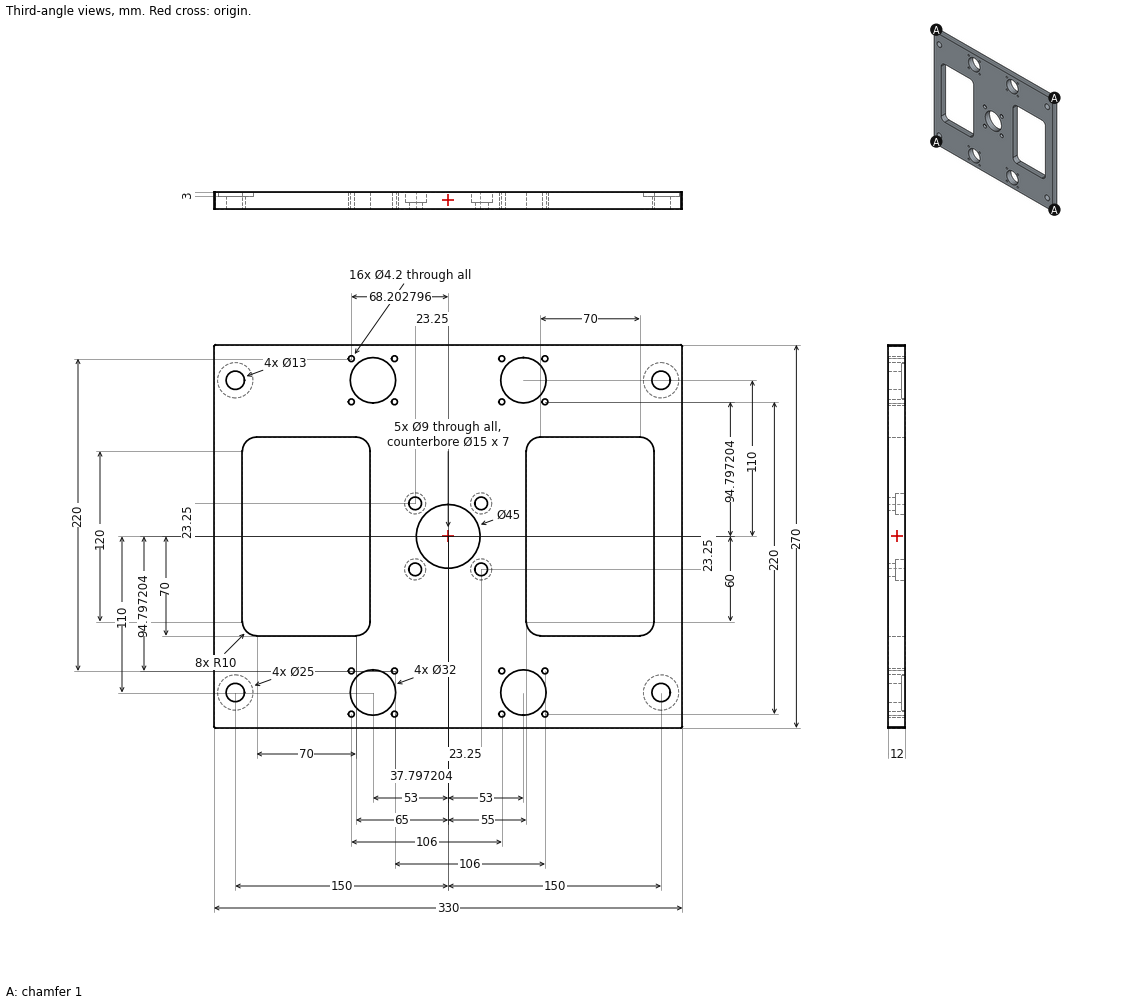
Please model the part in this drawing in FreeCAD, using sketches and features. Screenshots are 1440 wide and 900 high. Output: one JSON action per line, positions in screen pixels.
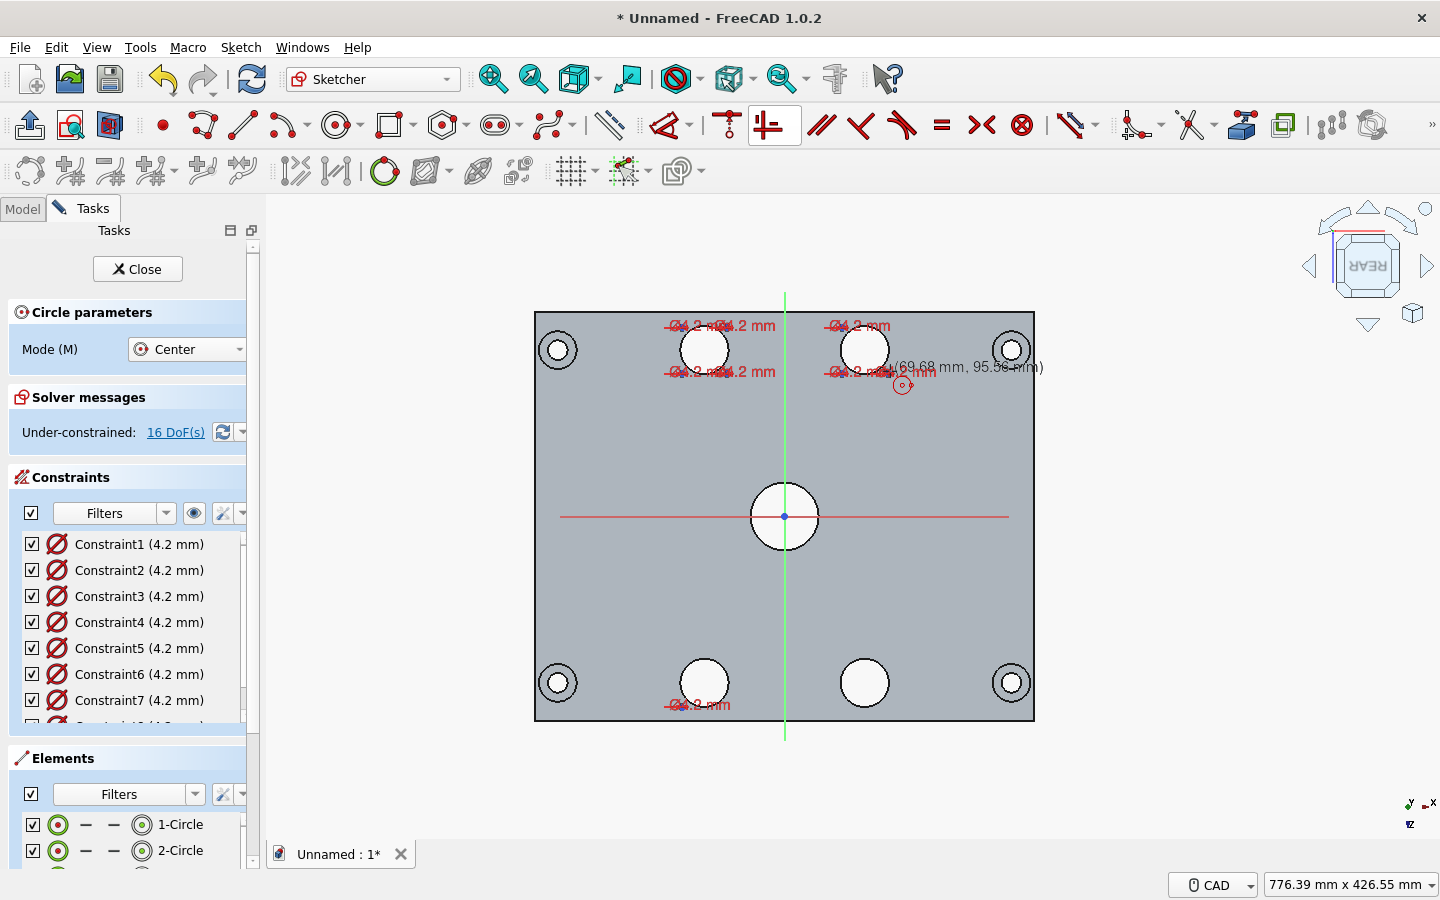
{"action": "scroll", "coordinate": [888, 327], "scroll_direction": "up", "scroll_amount": 10}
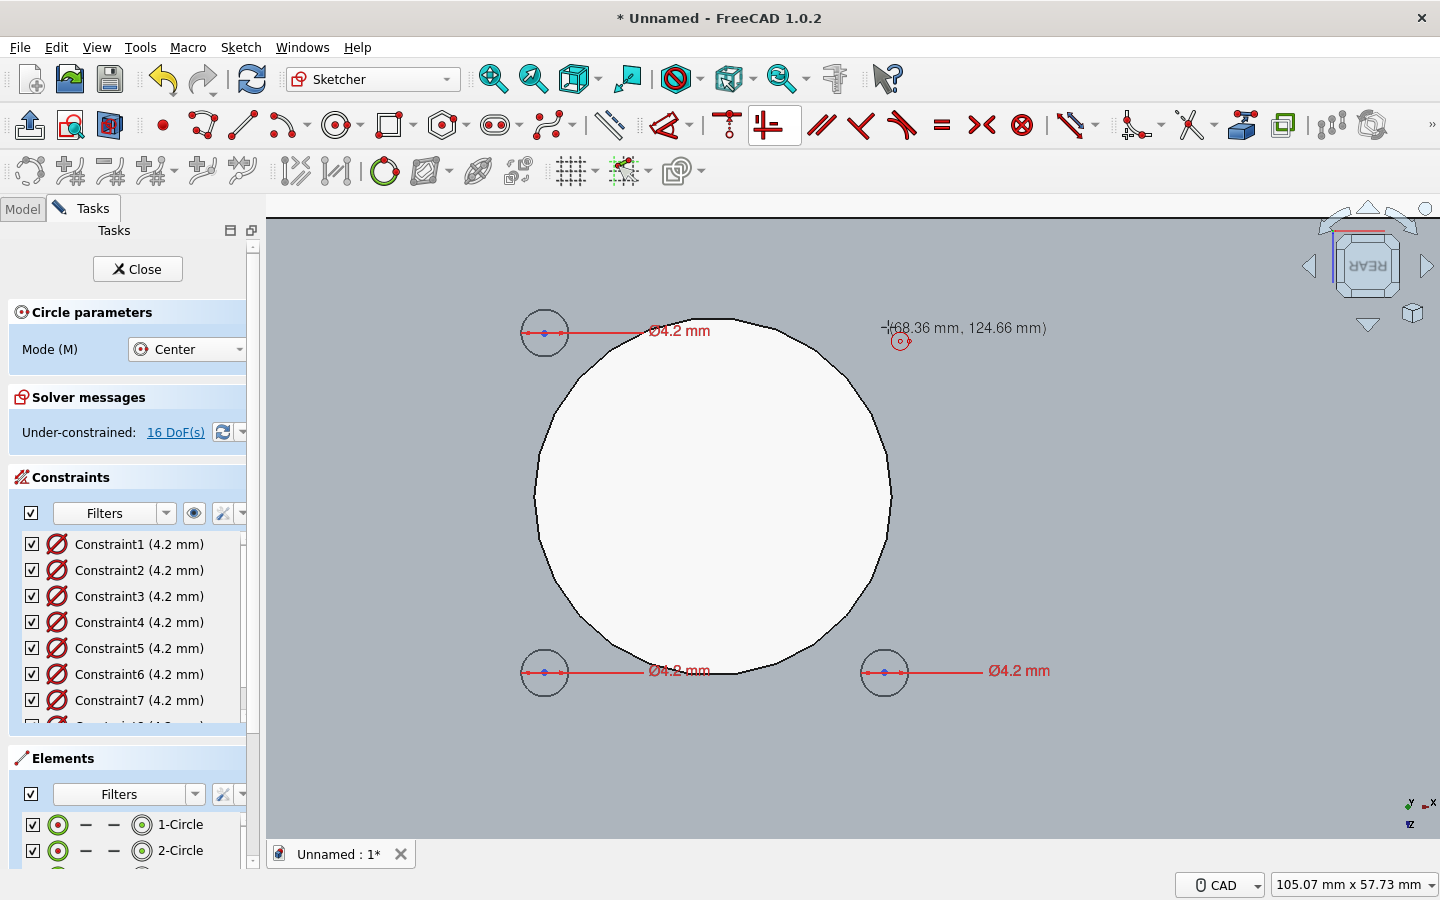
{"action": "scroll", "coordinate": [888, 327], "scroll_direction": "down", "scroll_amount": 10}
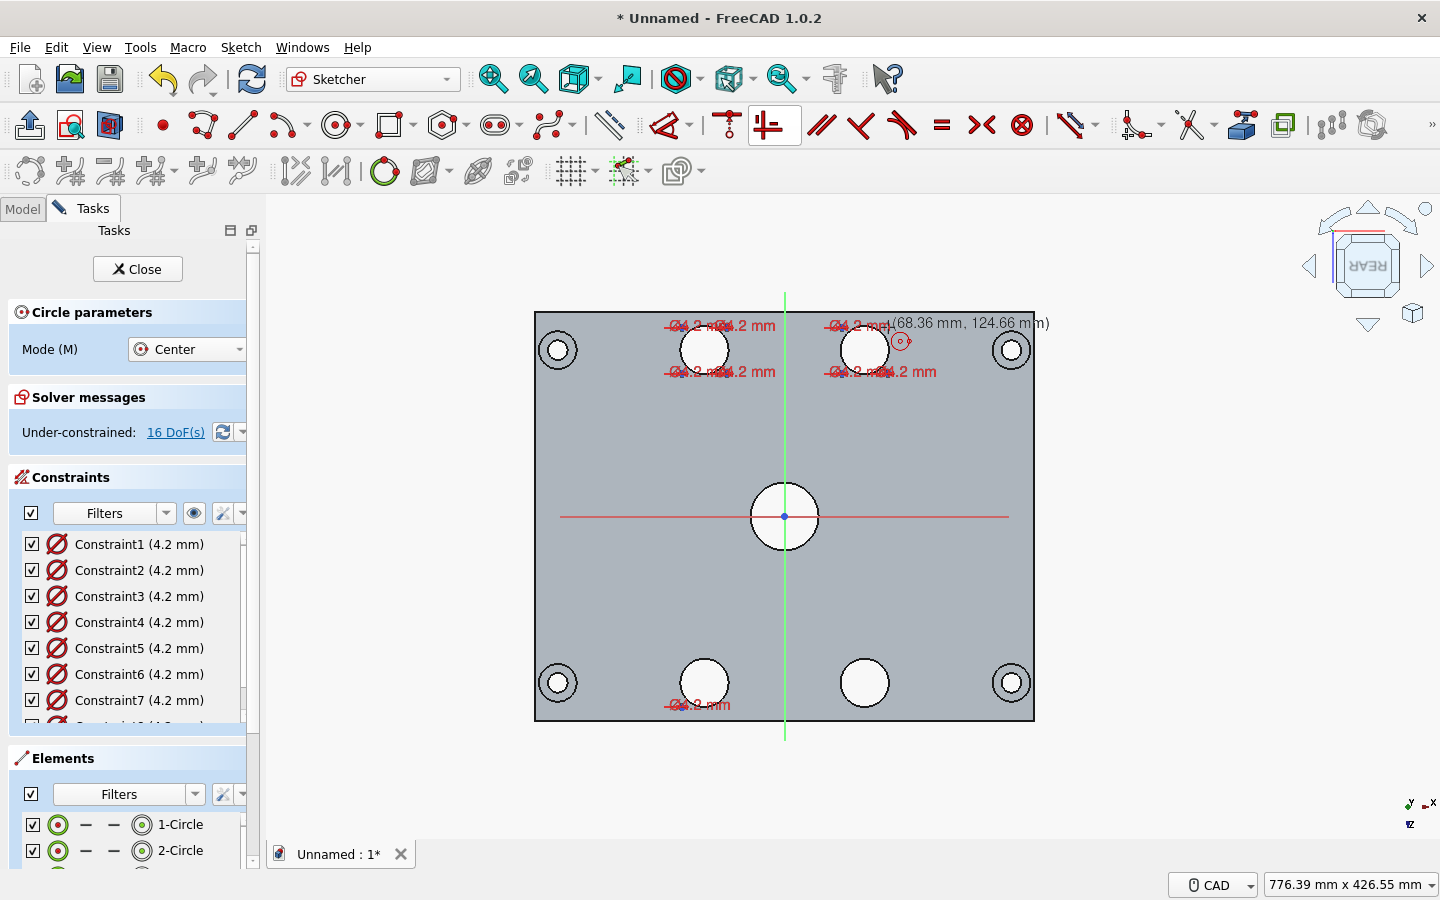
{"action": "left_click", "coordinate": [888, 327]}
{"action": "mouse_move", "coordinate": [890, 325]}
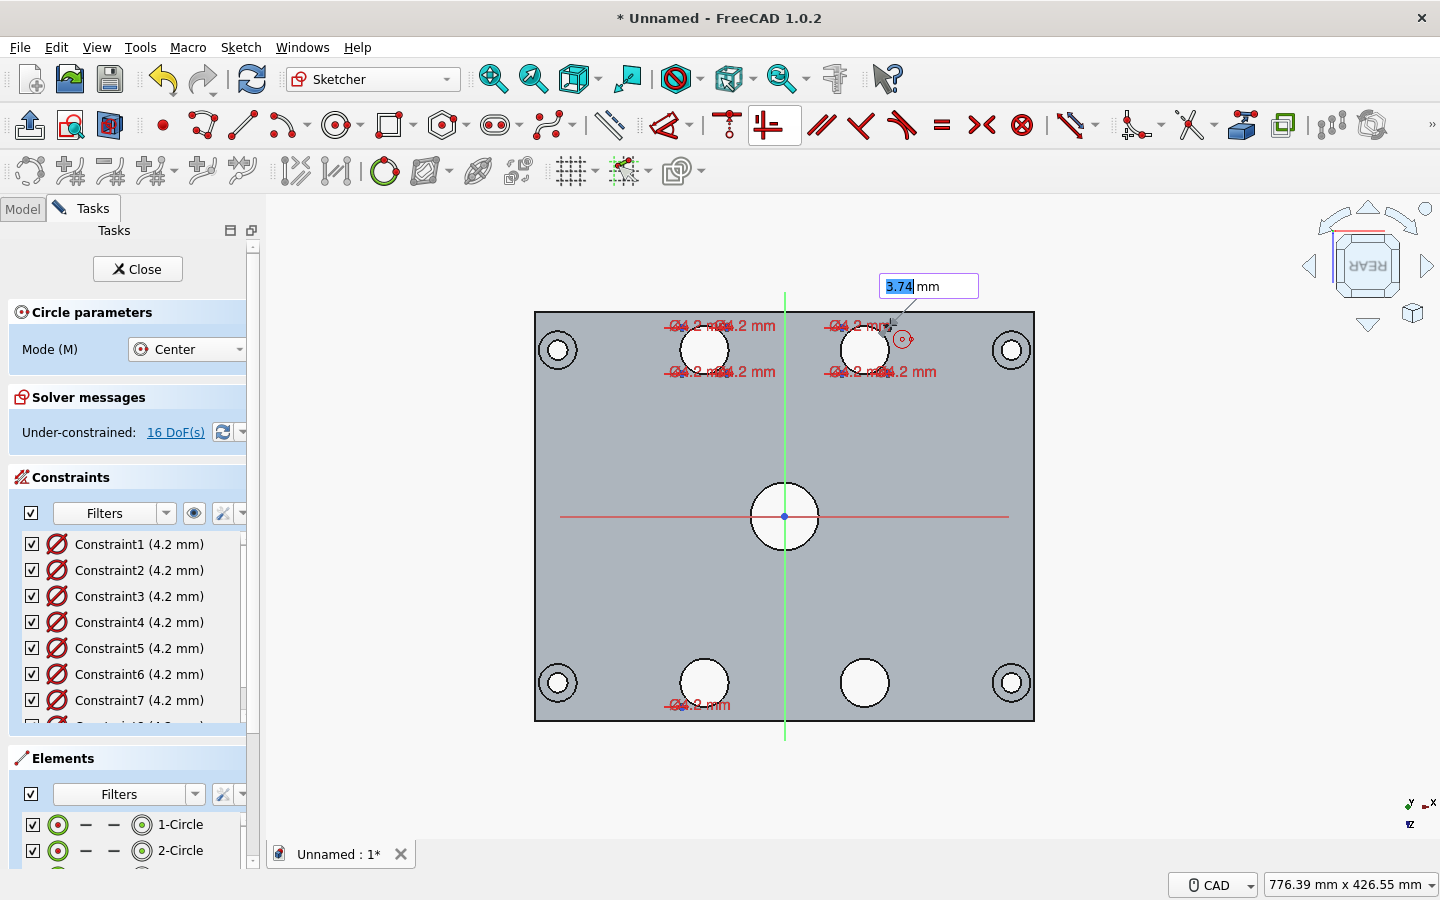
{"action": "type", "text": "4.2"}
{"action": "key", "text": "Return"}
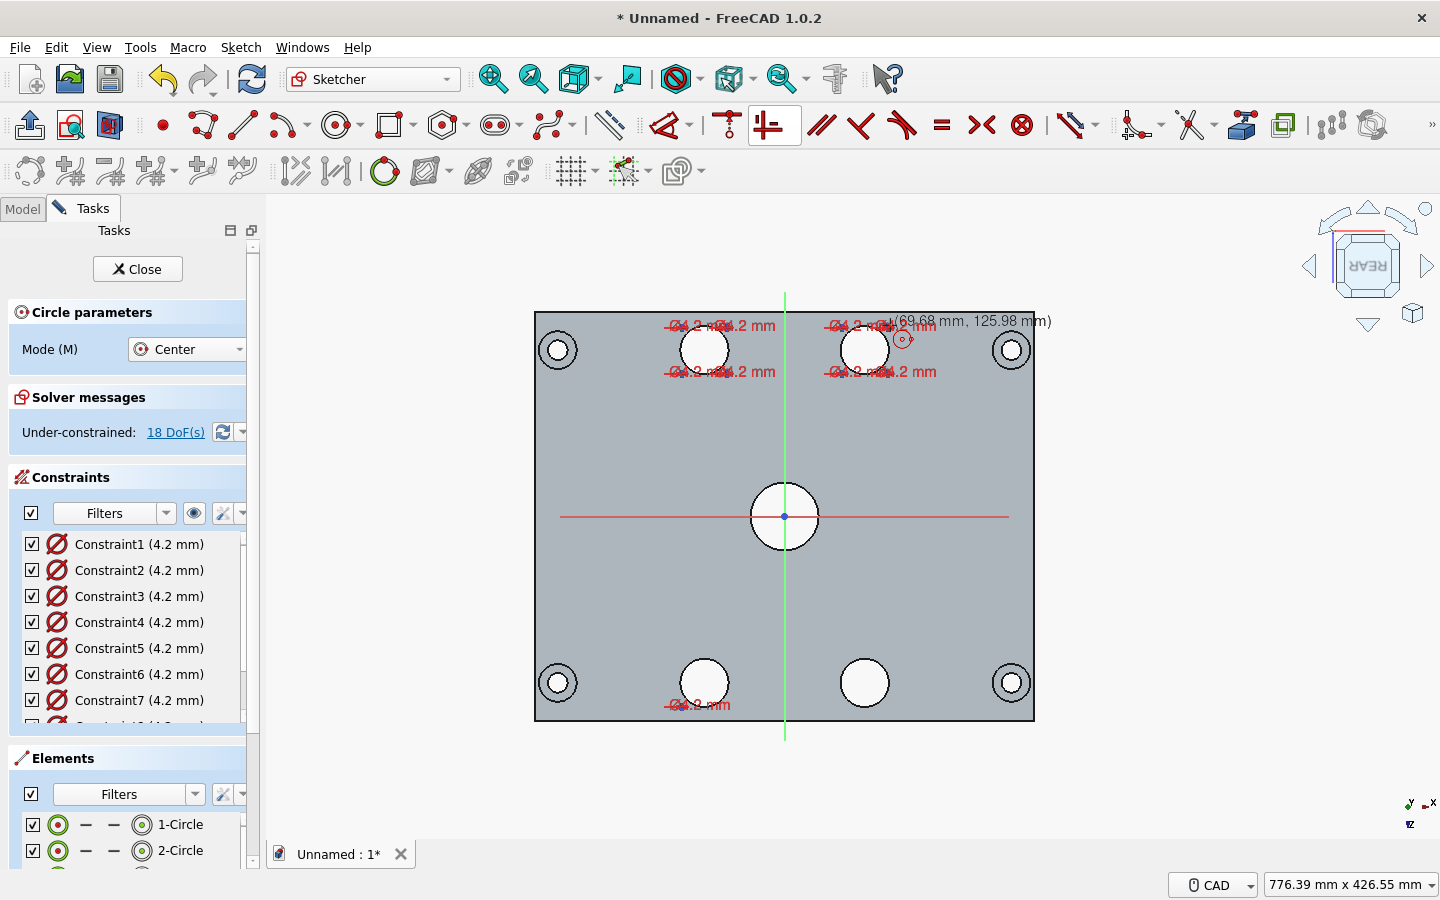
{"action": "scroll", "coordinate": [888, 706], "scroll_direction": "up", "scroll_amount": 10}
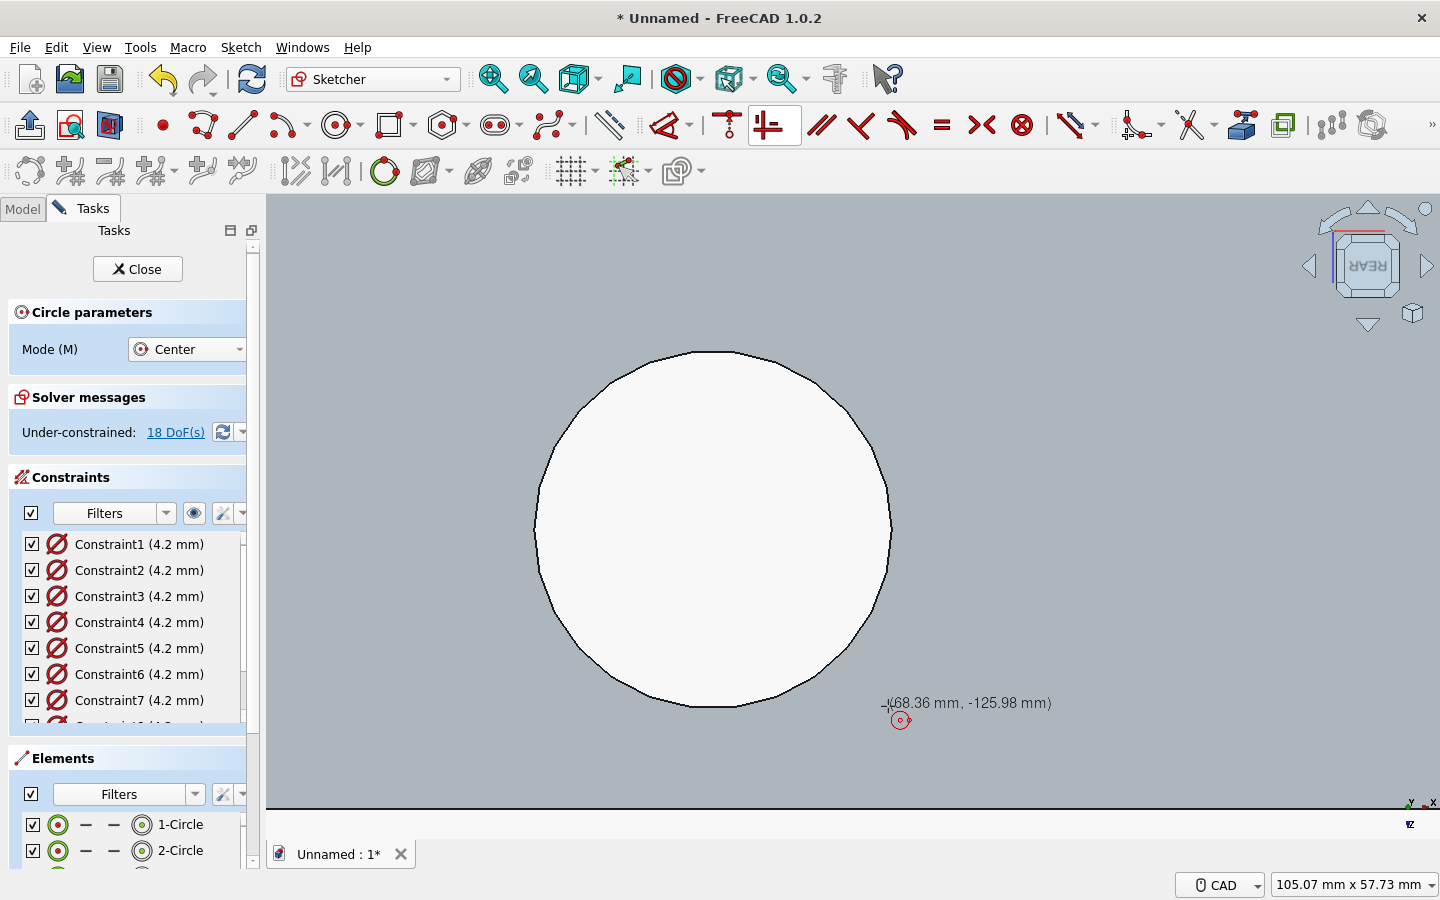
{"action": "scroll", "coordinate": [888, 707], "scroll_direction": "down", "scroll_amount": 10}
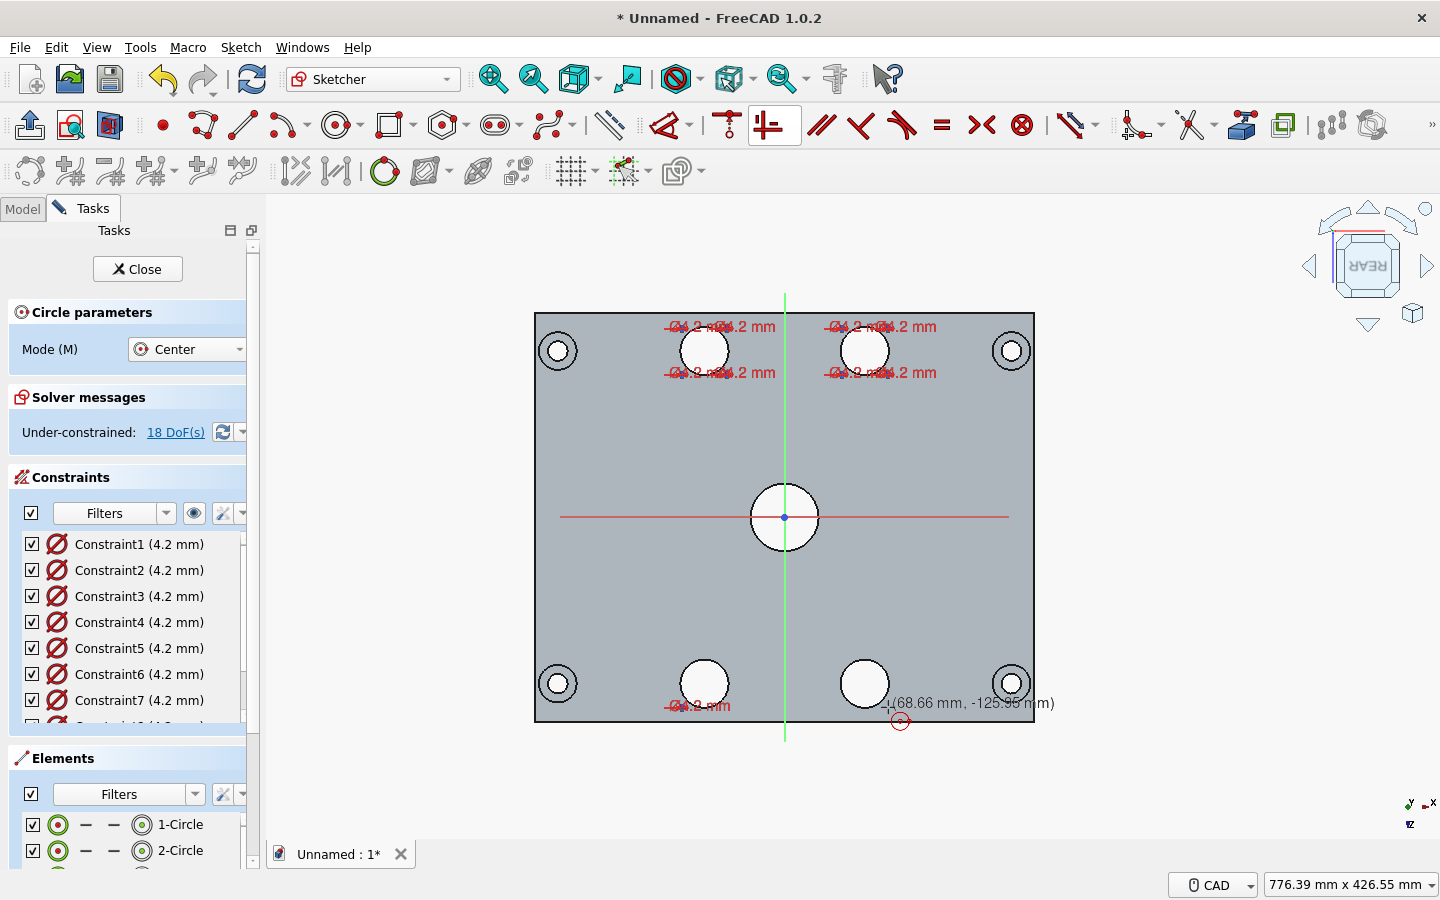
{"action": "left_click", "coordinate": [888, 707]}
{"action": "mouse_move", "coordinate": [890, 704]}